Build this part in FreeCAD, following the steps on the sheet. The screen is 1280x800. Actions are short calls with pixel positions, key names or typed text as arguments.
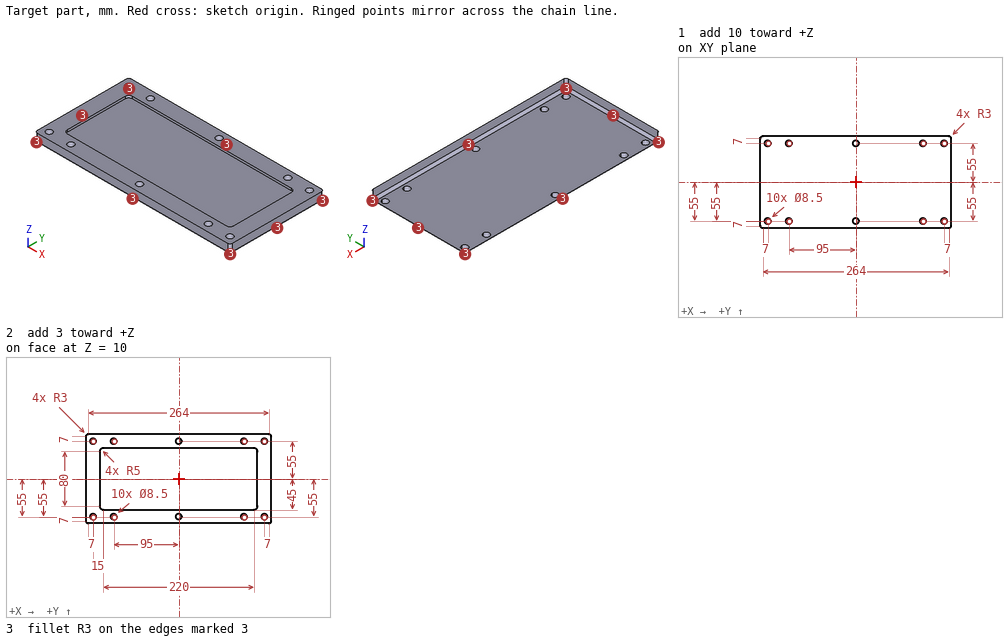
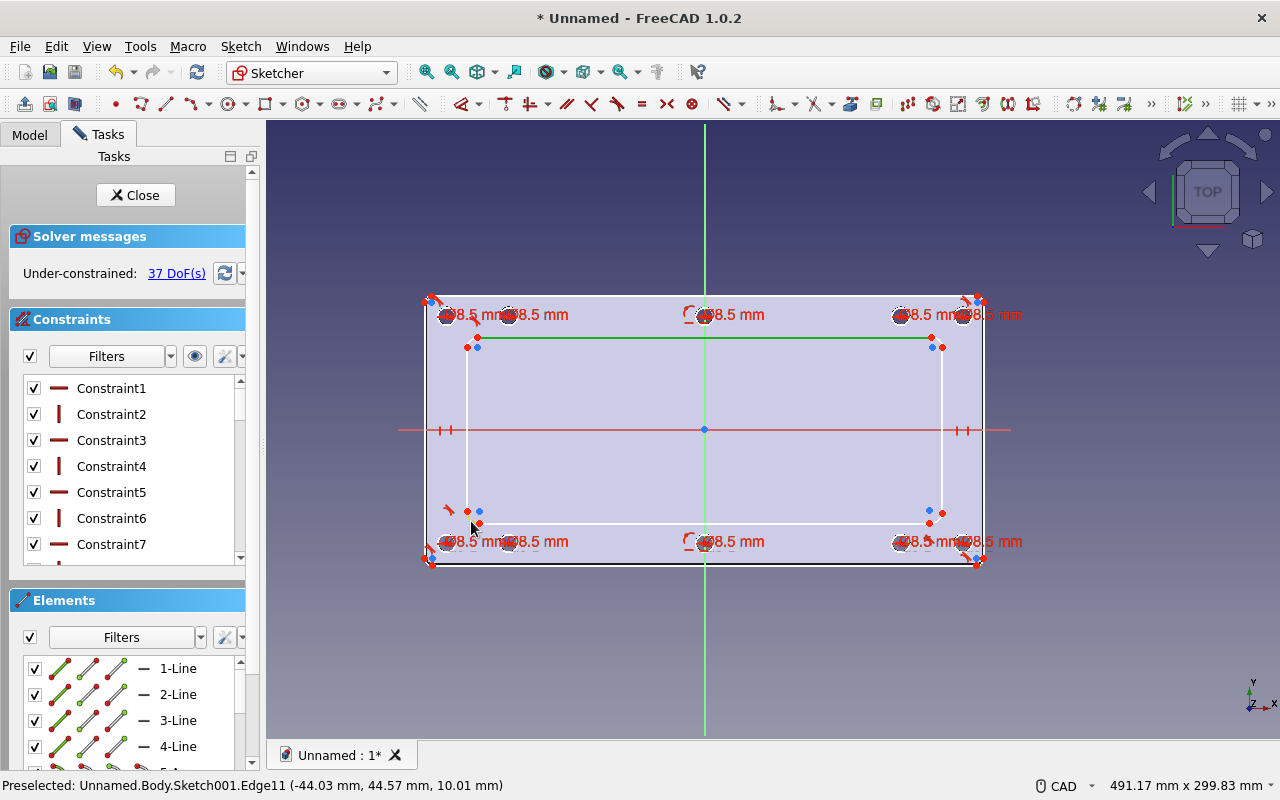
scroll(941, 343, up, 6)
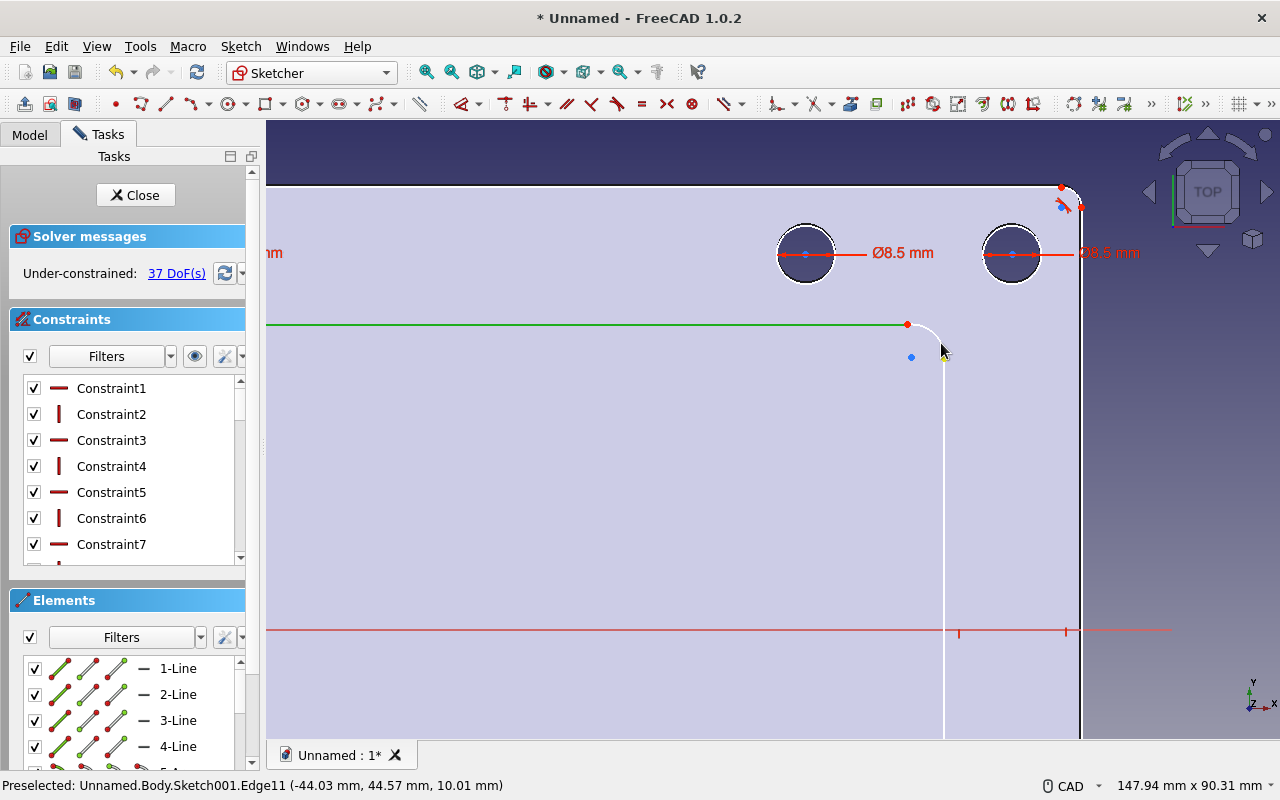
click(940, 342)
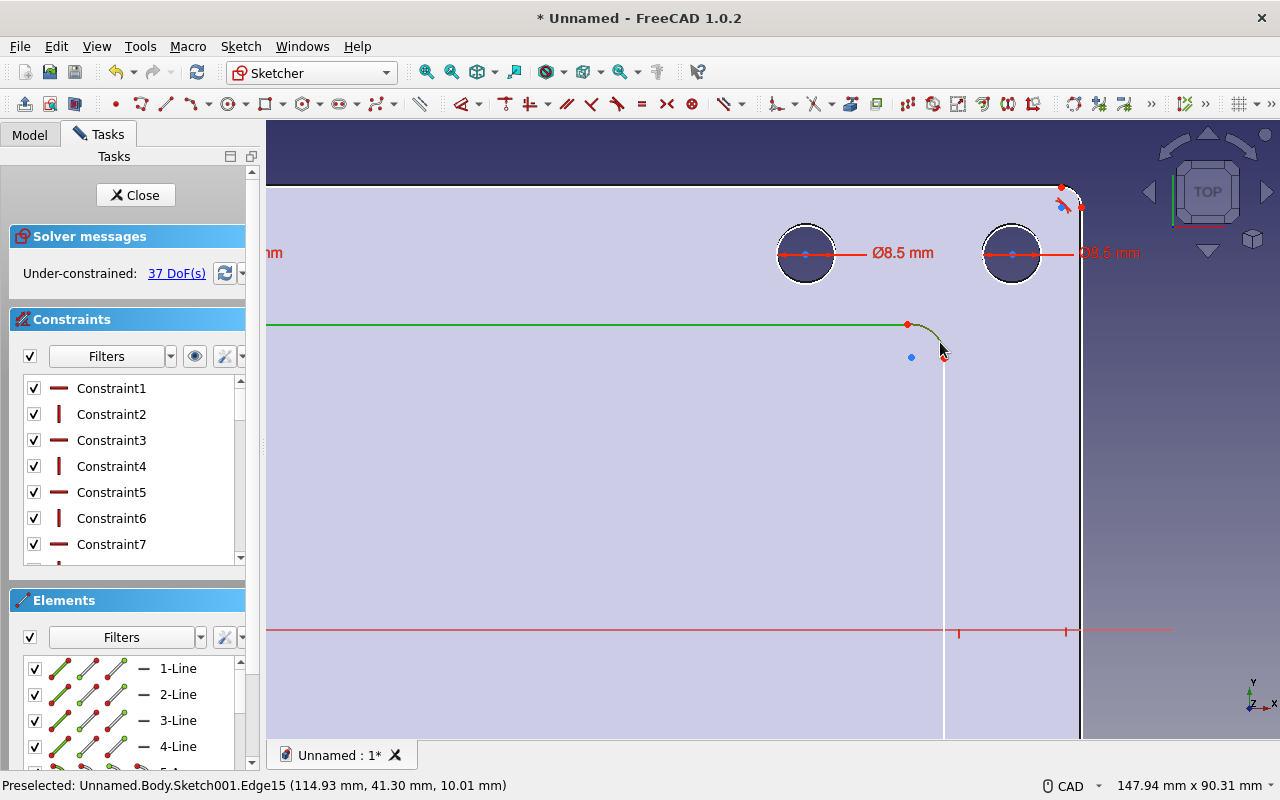
click(617, 104)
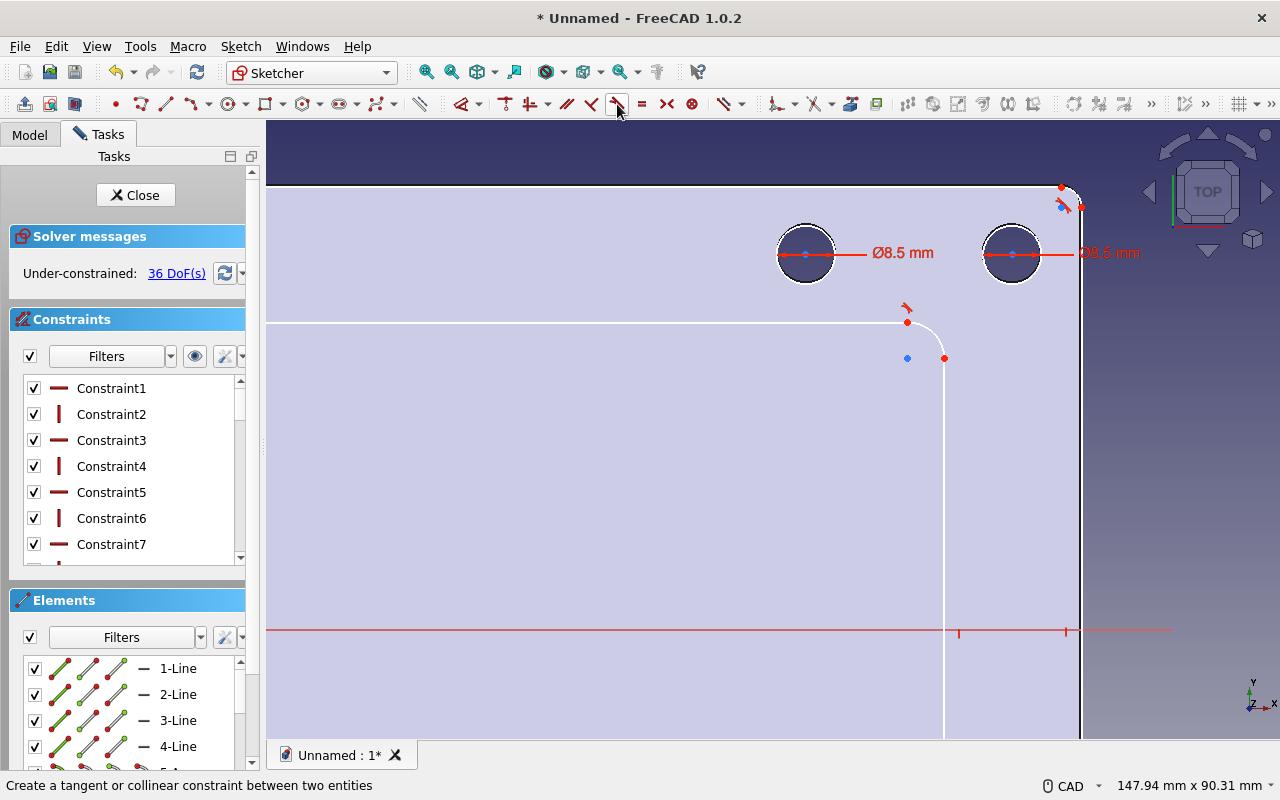
click(944, 523)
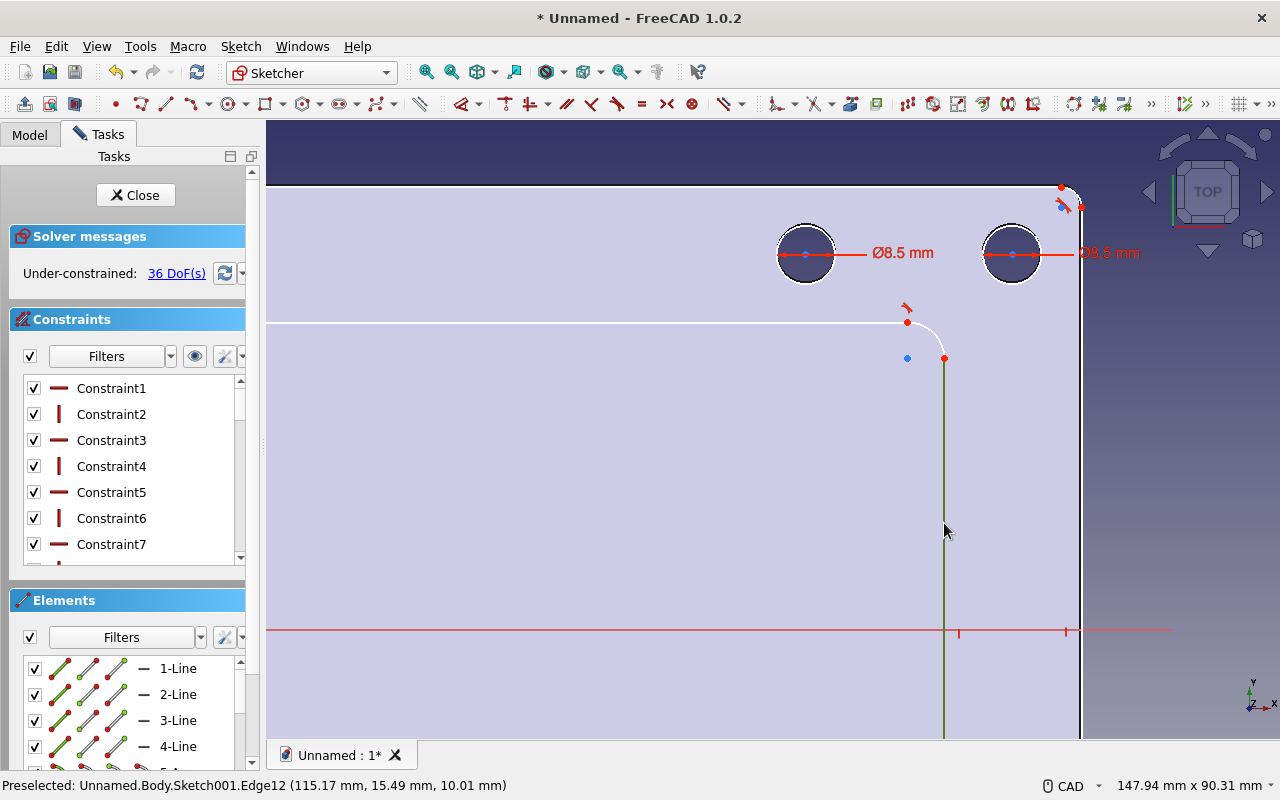
click(940, 342)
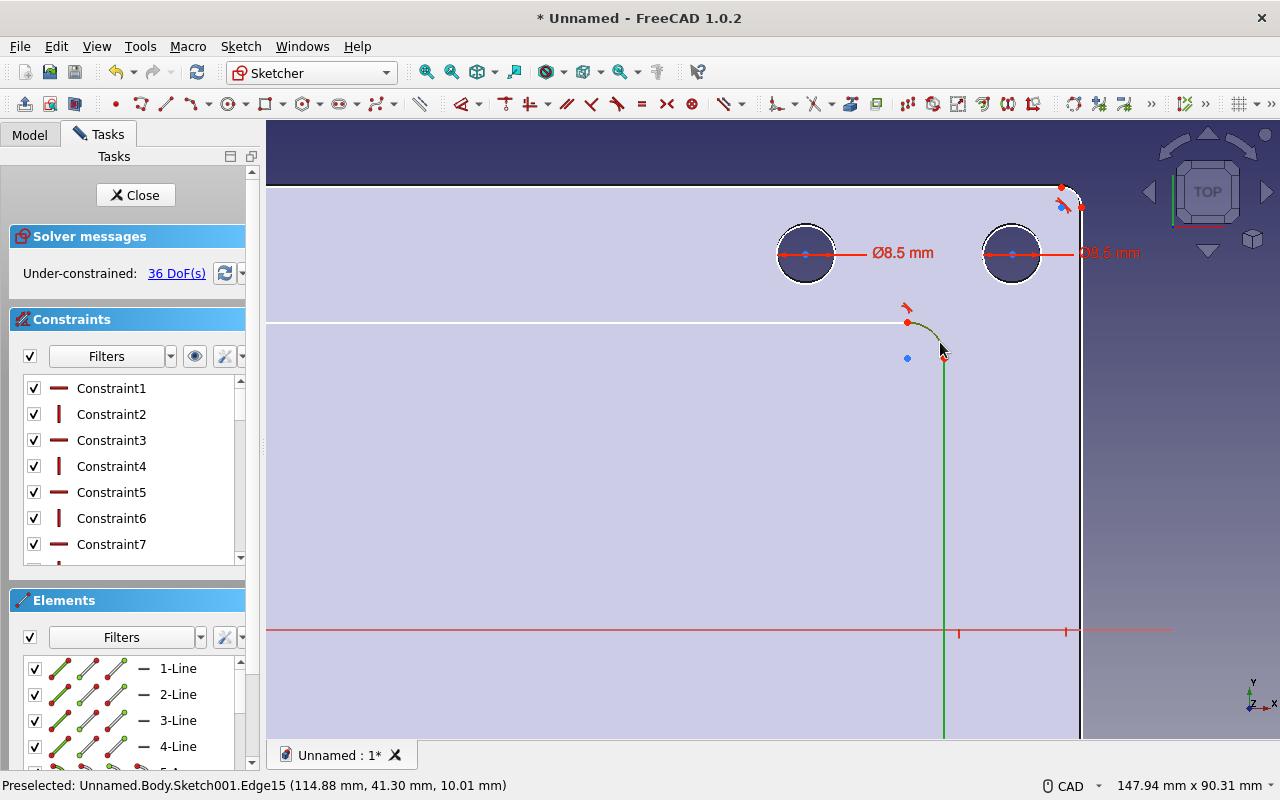
click(617, 104)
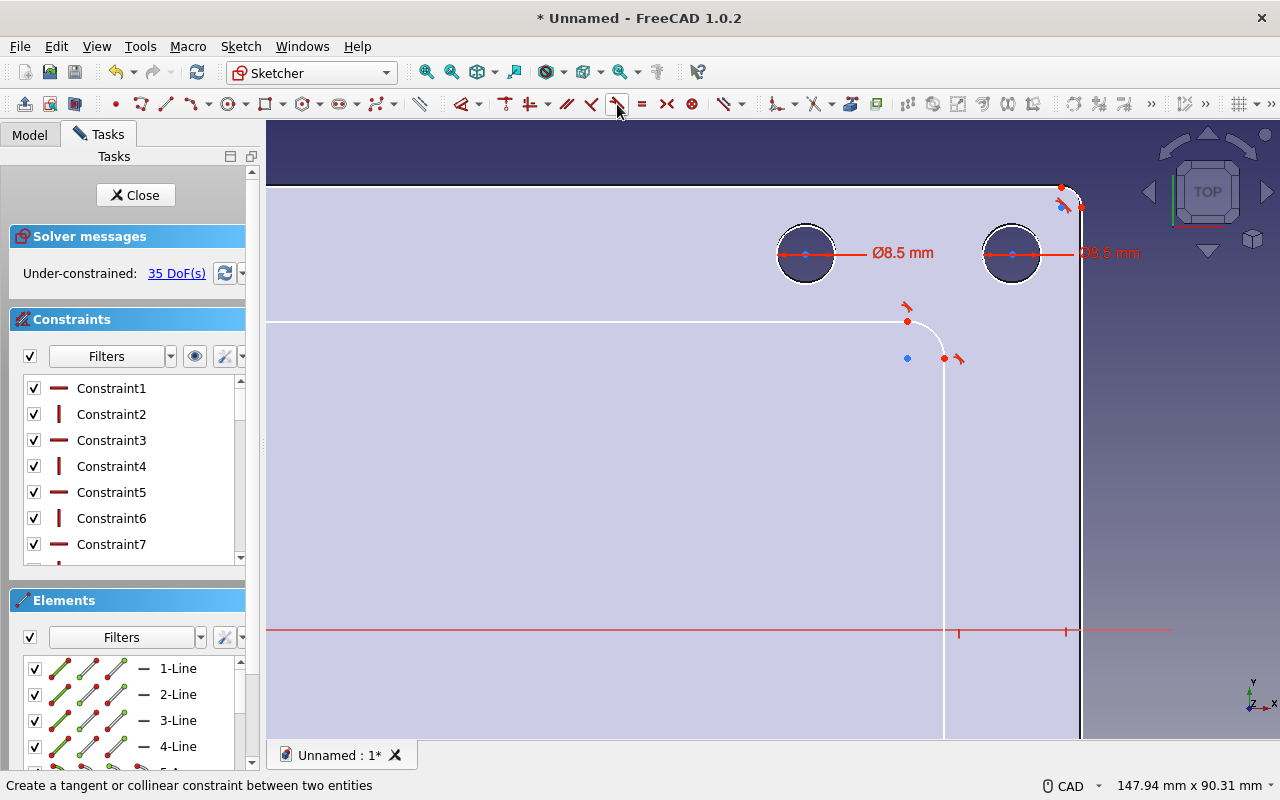
click(944, 523)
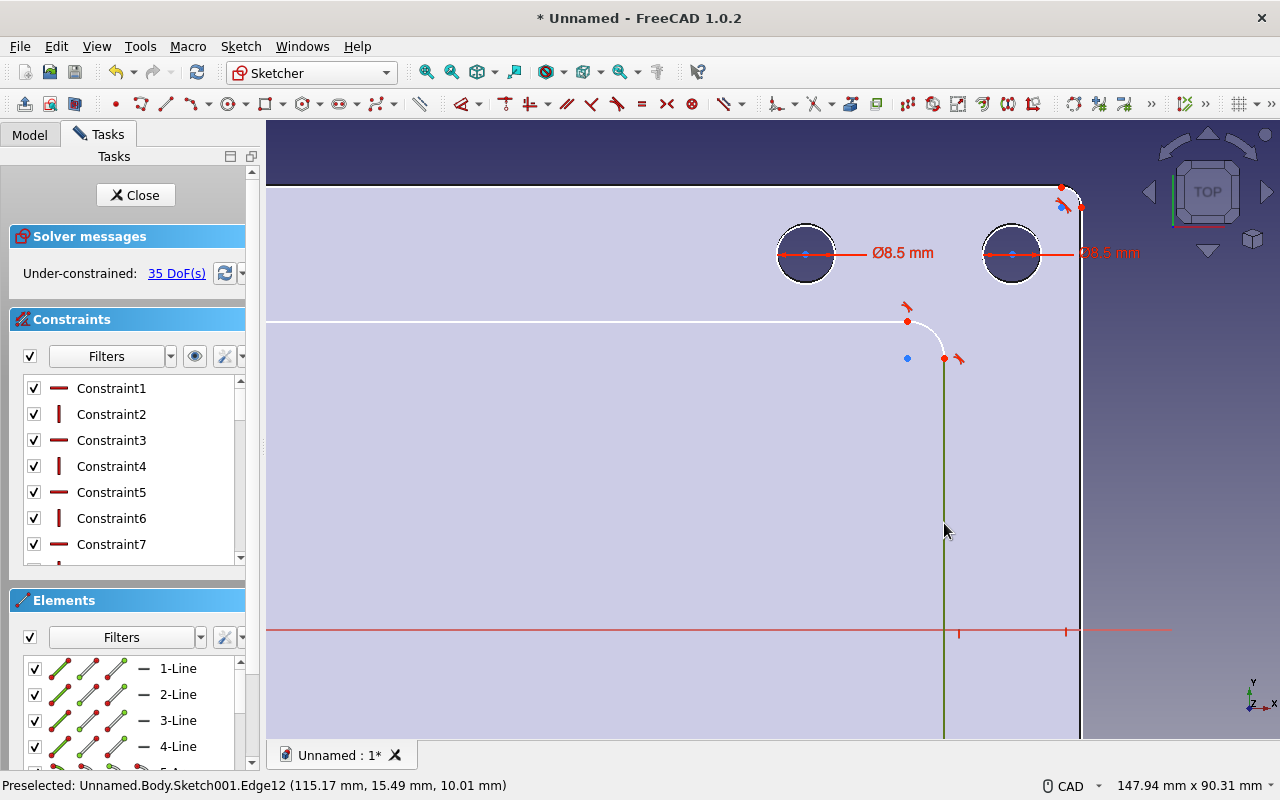
scroll(941, 343, down, 6)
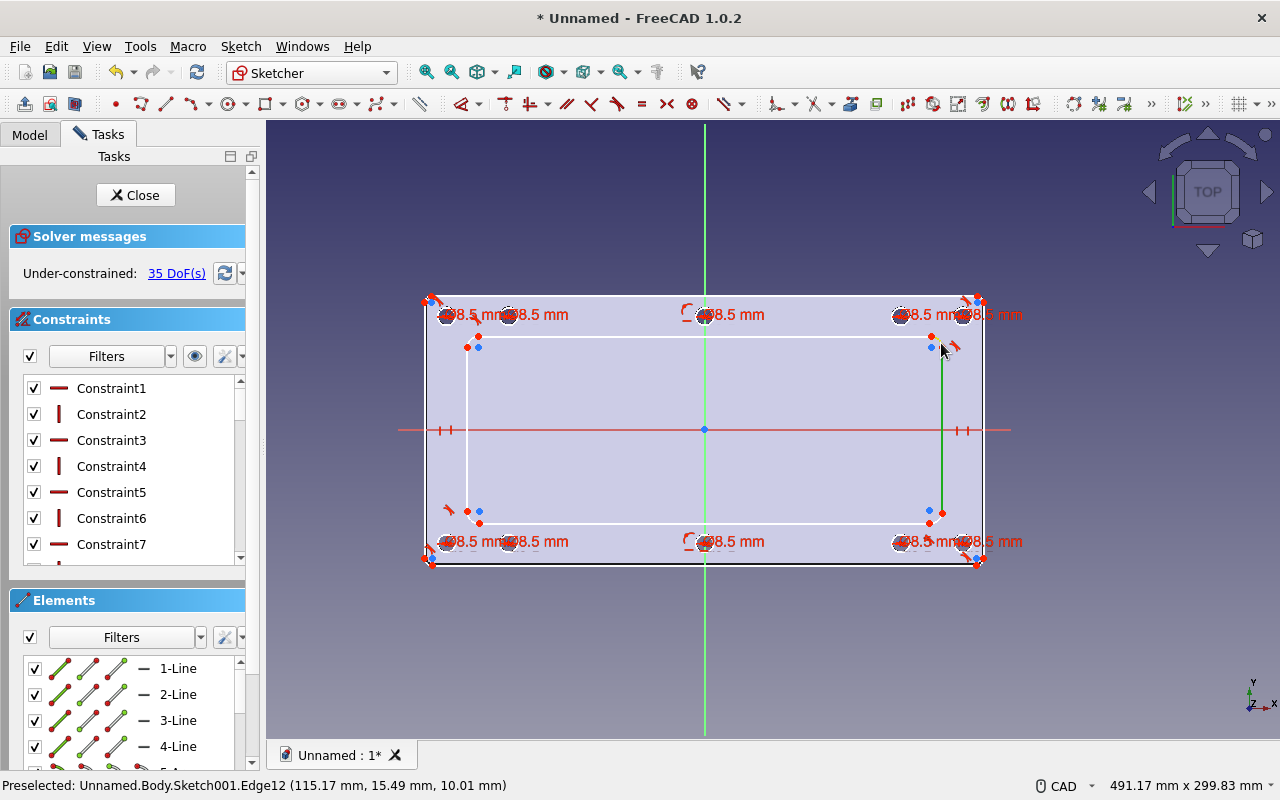
scroll(934, 523, up, 5)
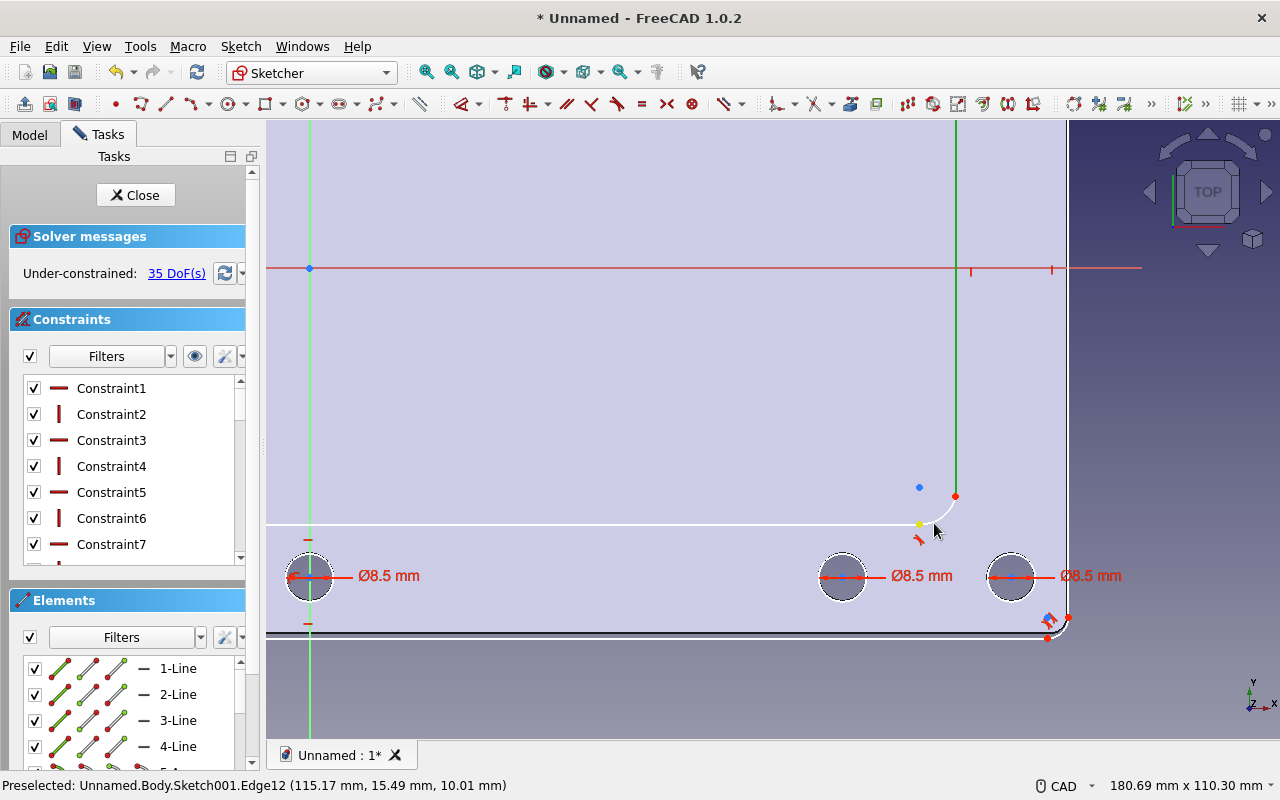
click(934, 522)